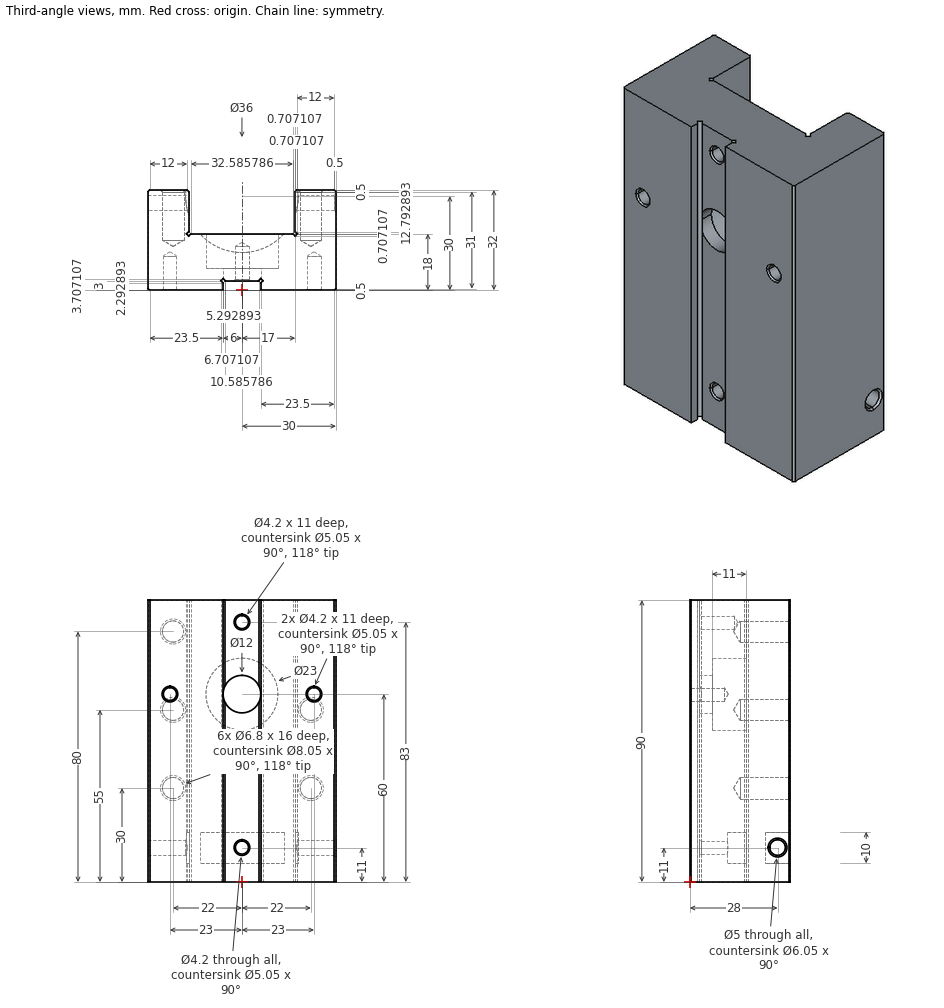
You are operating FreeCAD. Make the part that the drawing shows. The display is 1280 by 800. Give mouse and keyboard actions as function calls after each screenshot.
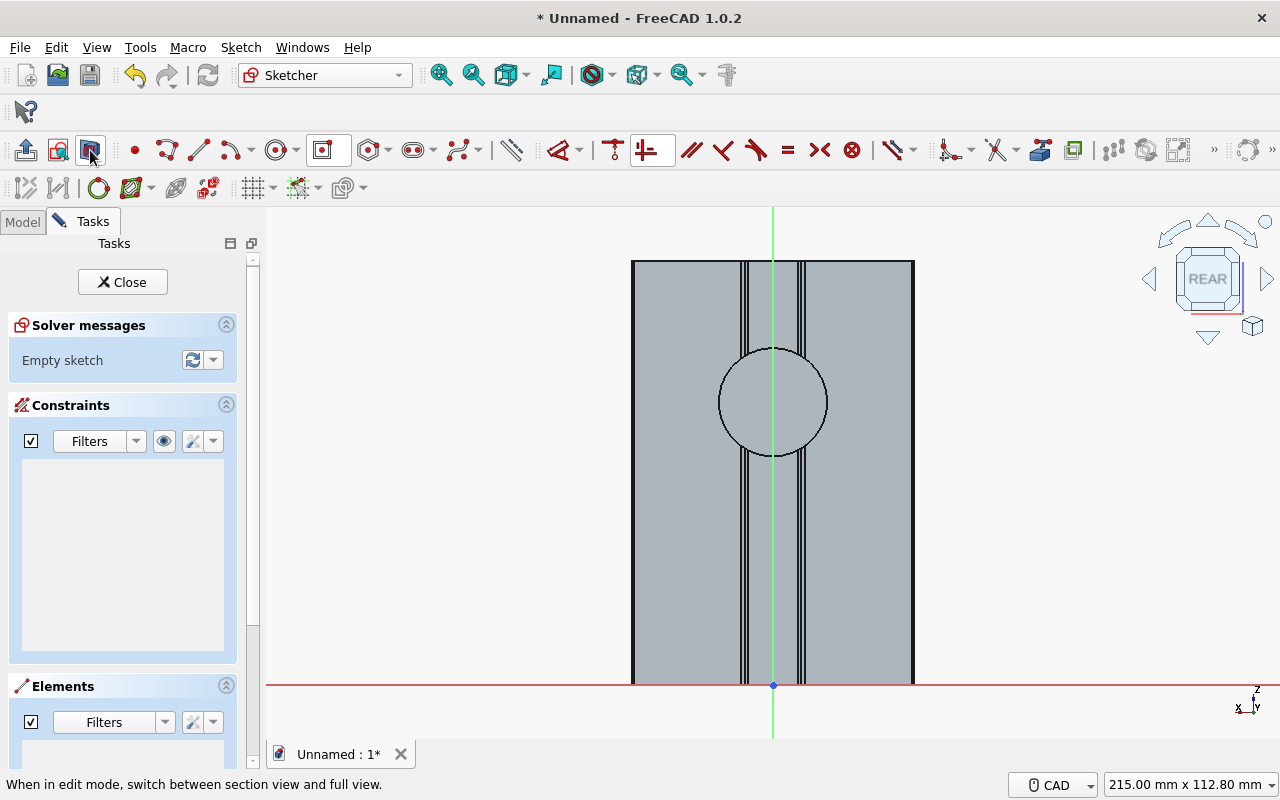
scroll(787, 388, up, 9)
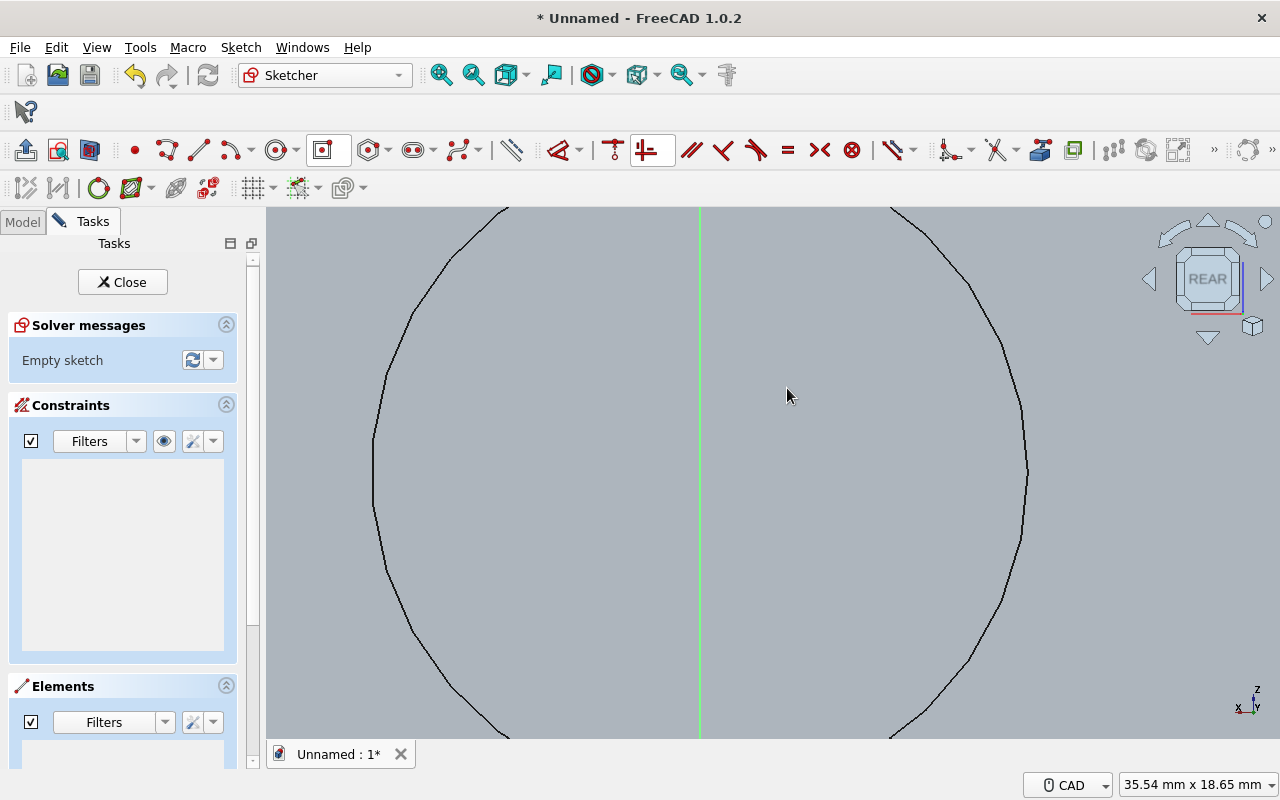
click(276, 150)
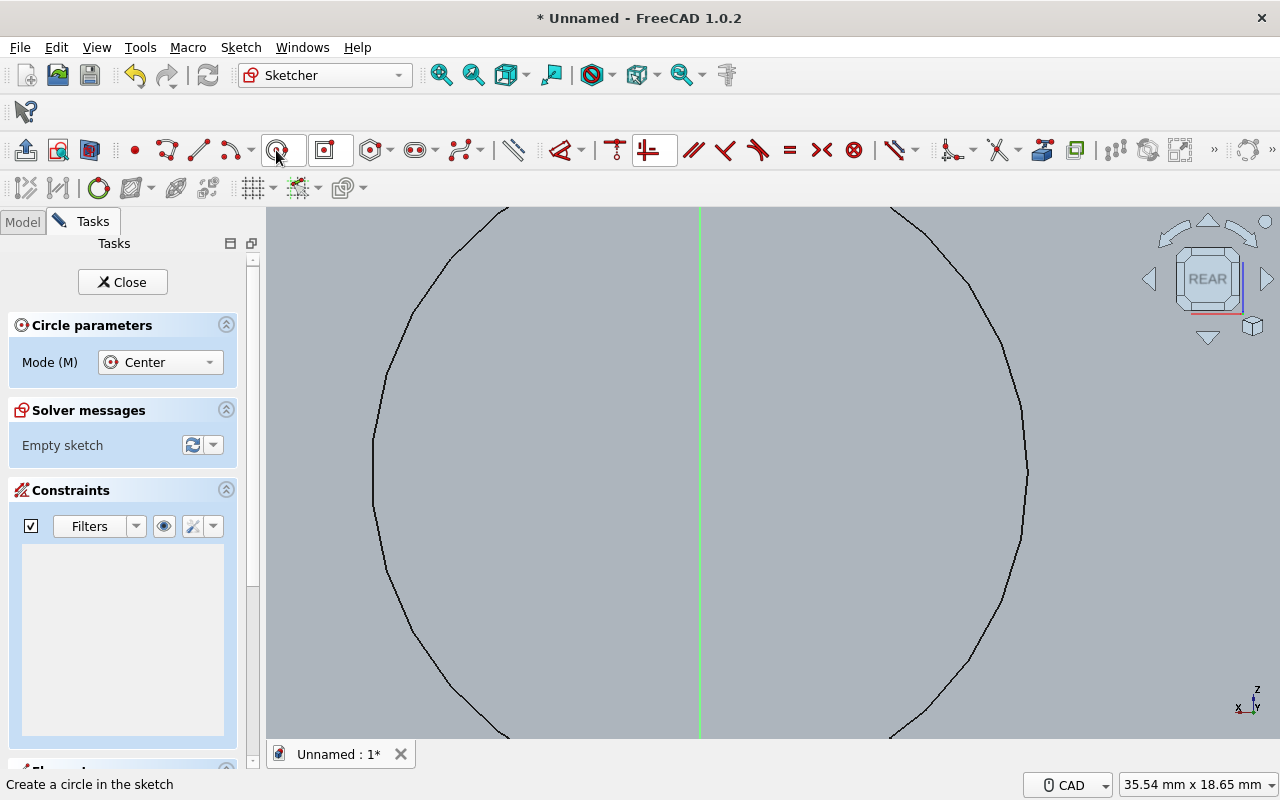
click(700, 473)
move(821, 351)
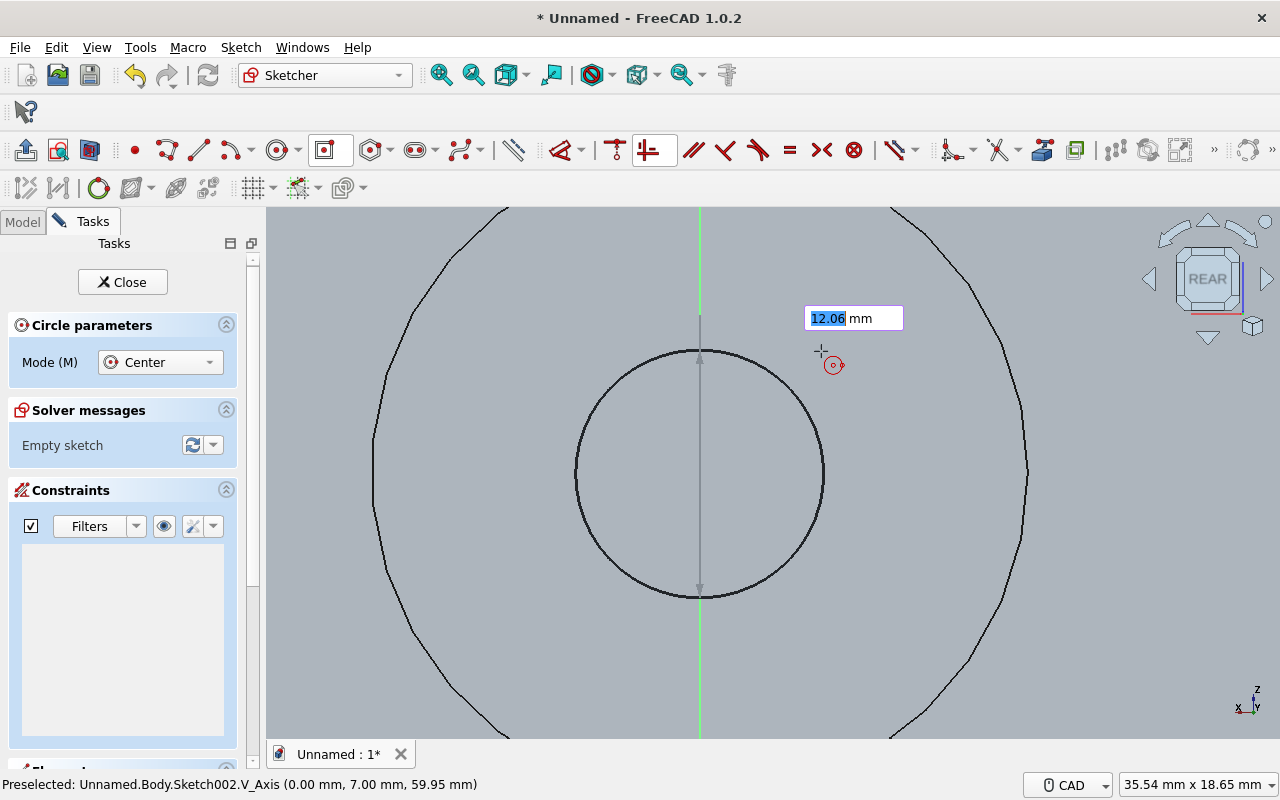
text(12)
key(Return)
key(Escape)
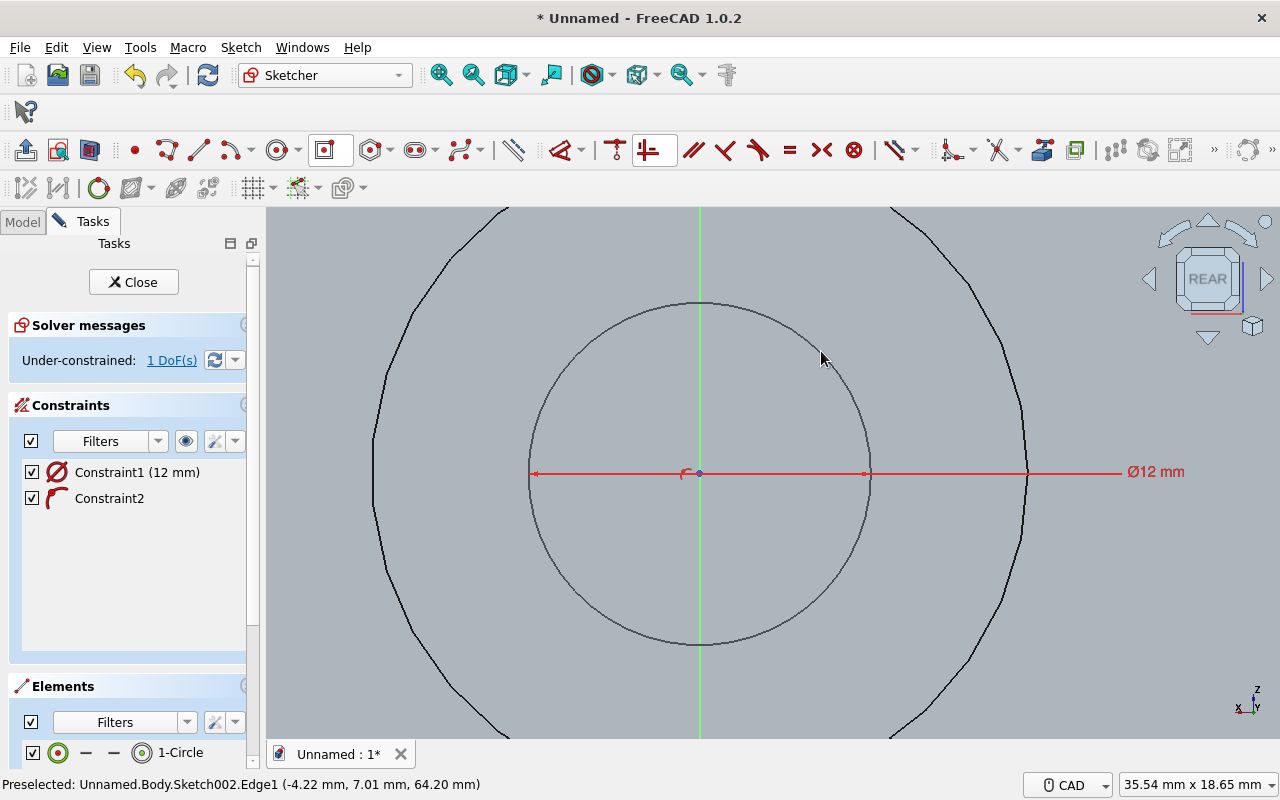
click(560, 150)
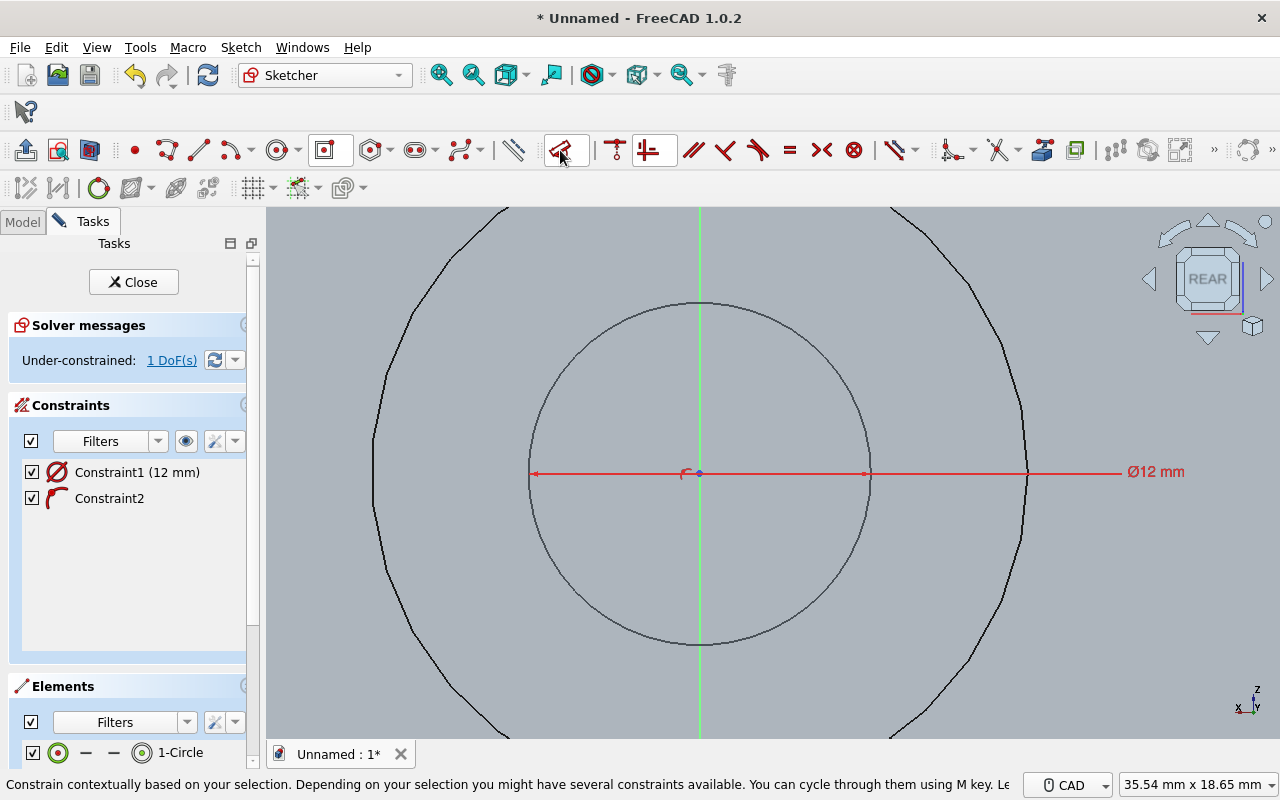
click(700, 474)
click(734, 593)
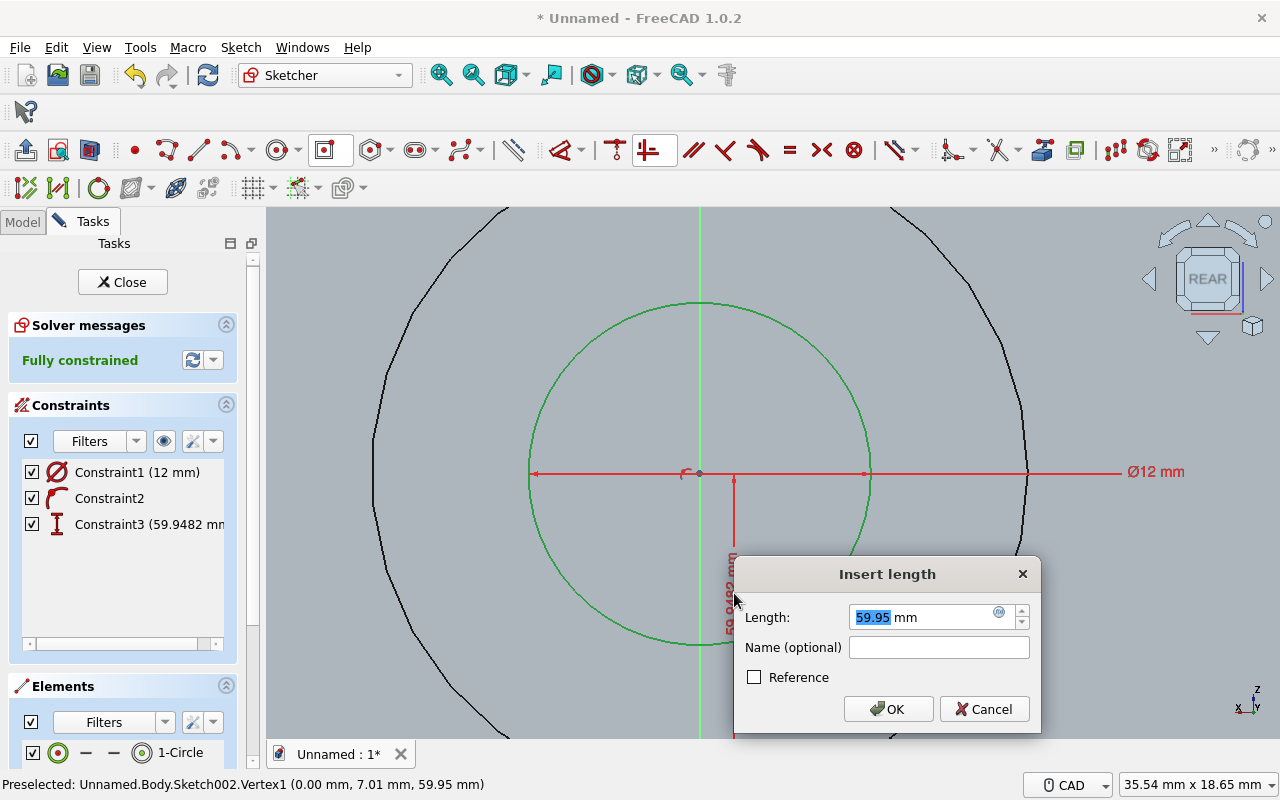
text(60)
key(Return)
key(Escape)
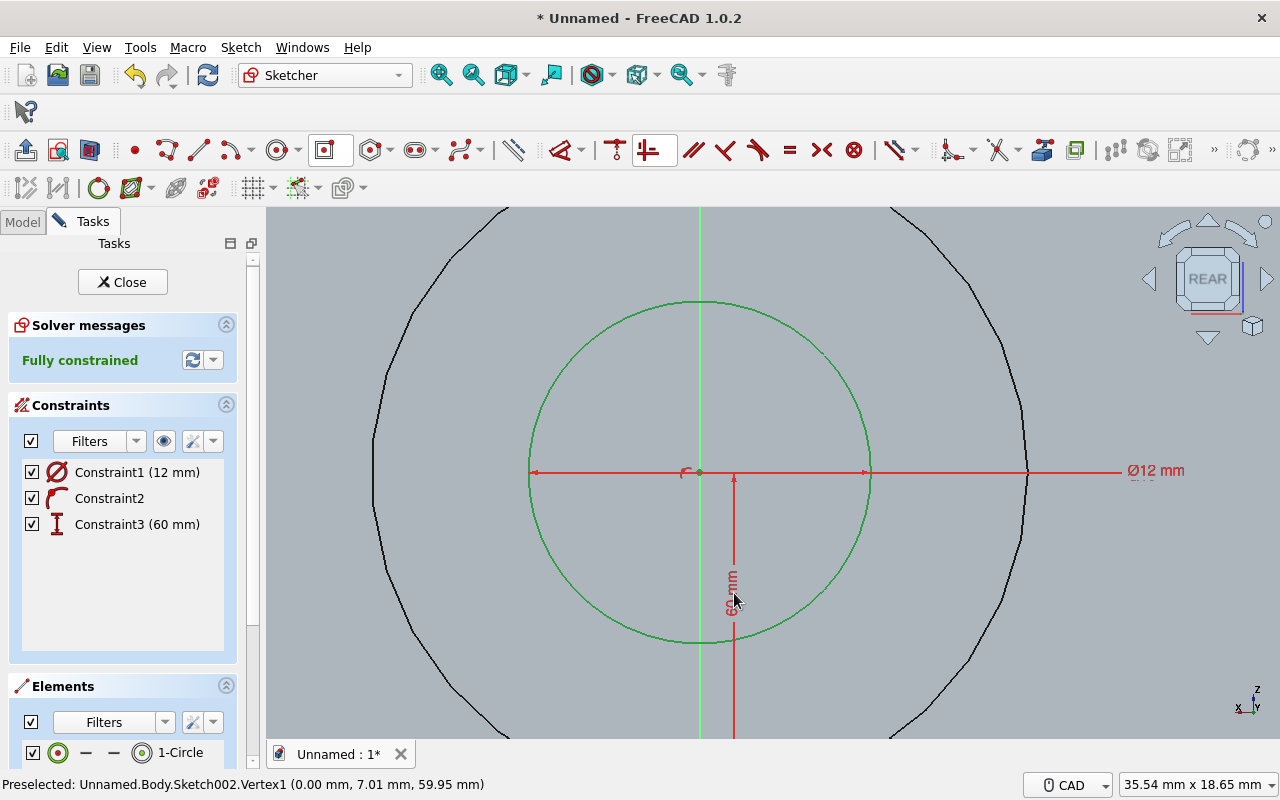
click(123, 282)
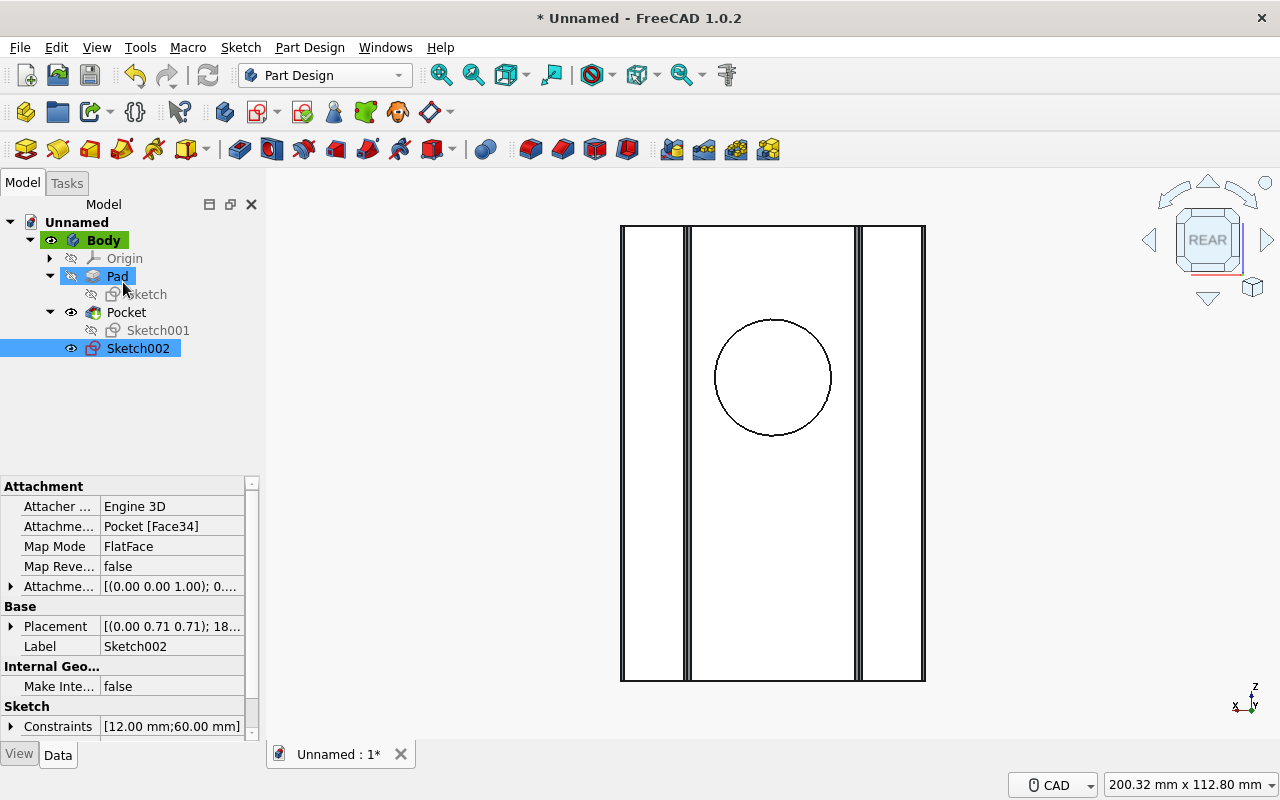
click(240, 150)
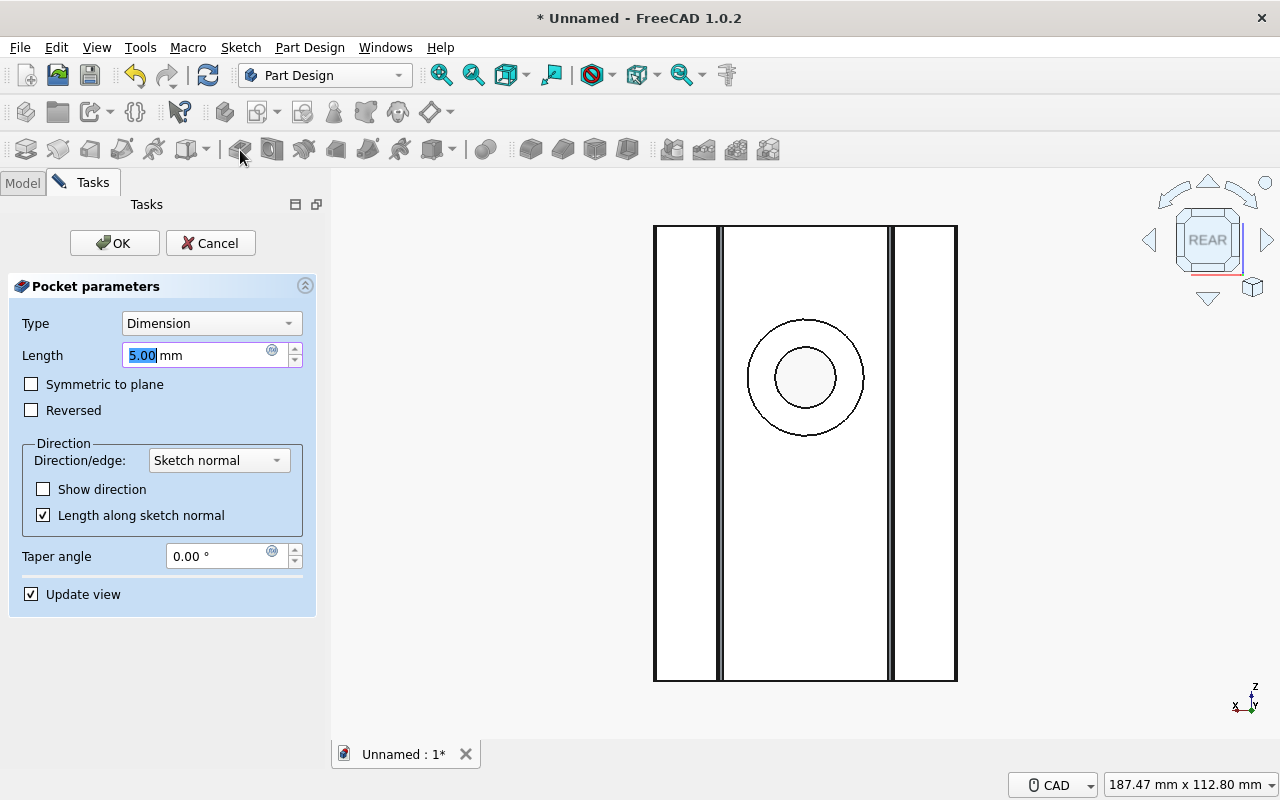
click(212, 324)